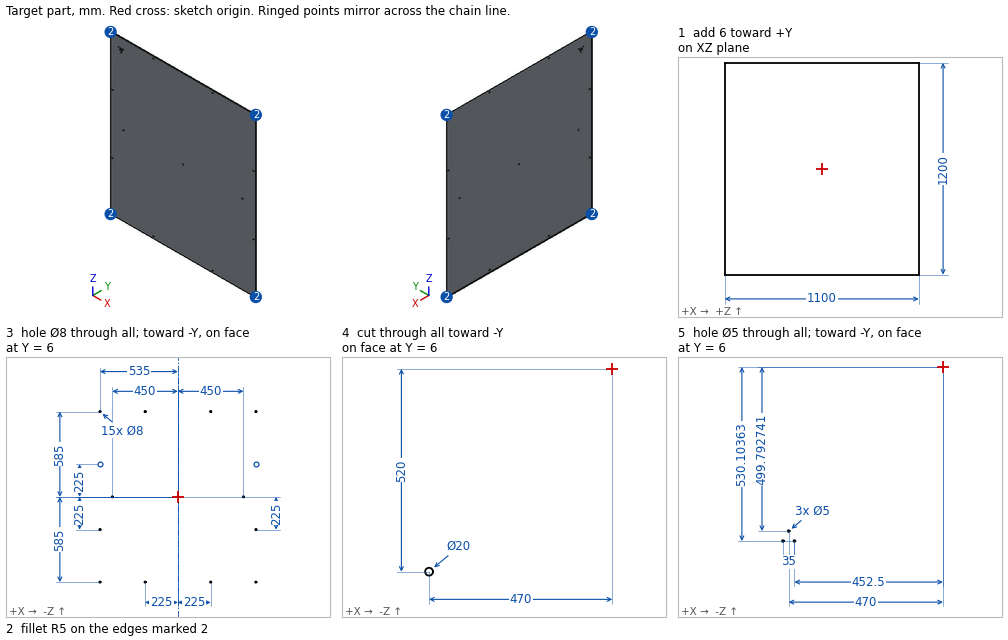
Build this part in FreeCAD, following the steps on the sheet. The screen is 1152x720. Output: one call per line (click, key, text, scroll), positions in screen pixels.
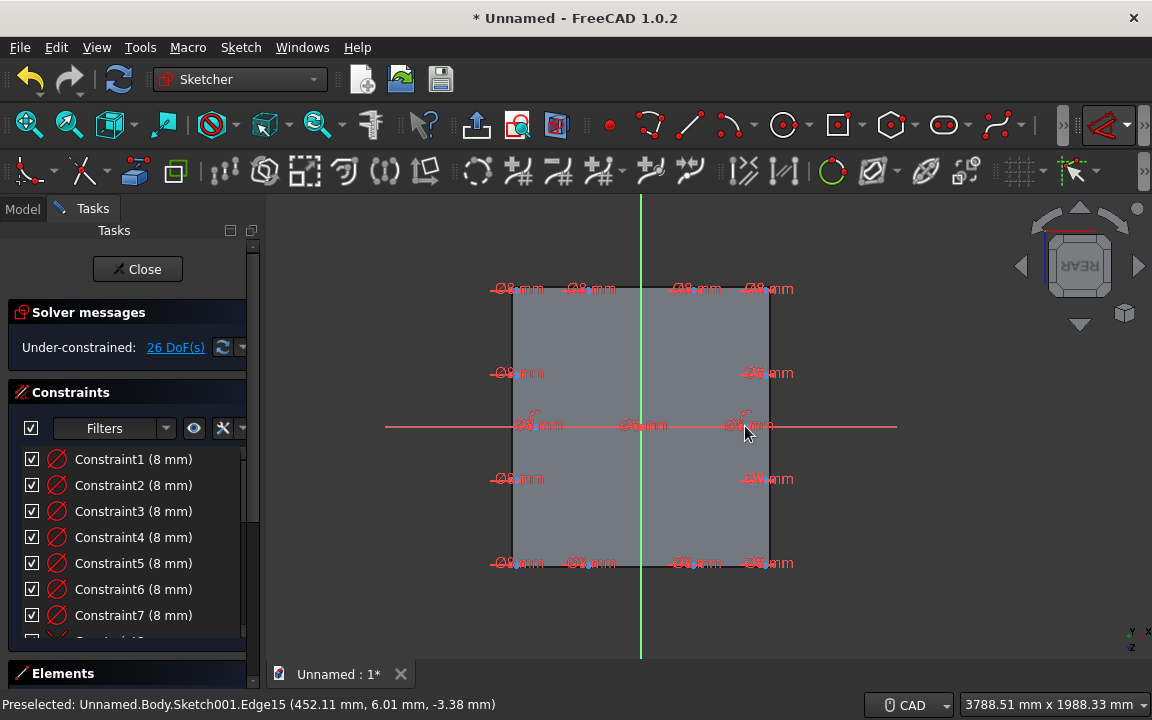
click(516, 291)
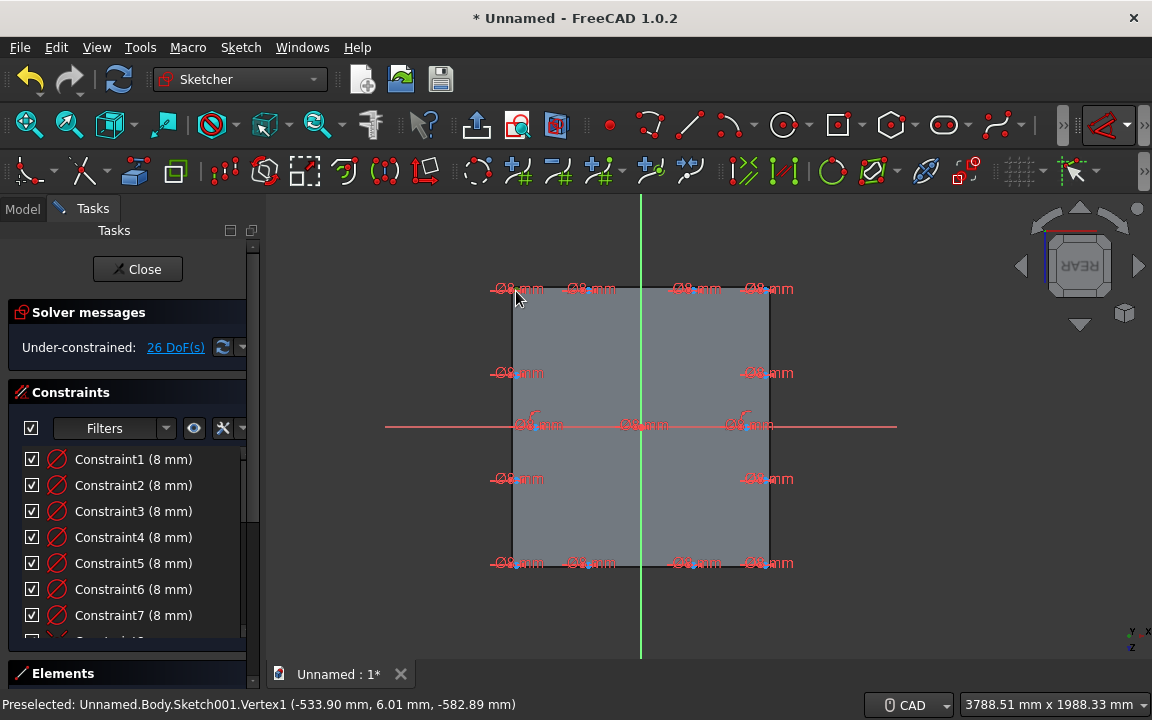
click(766, 291)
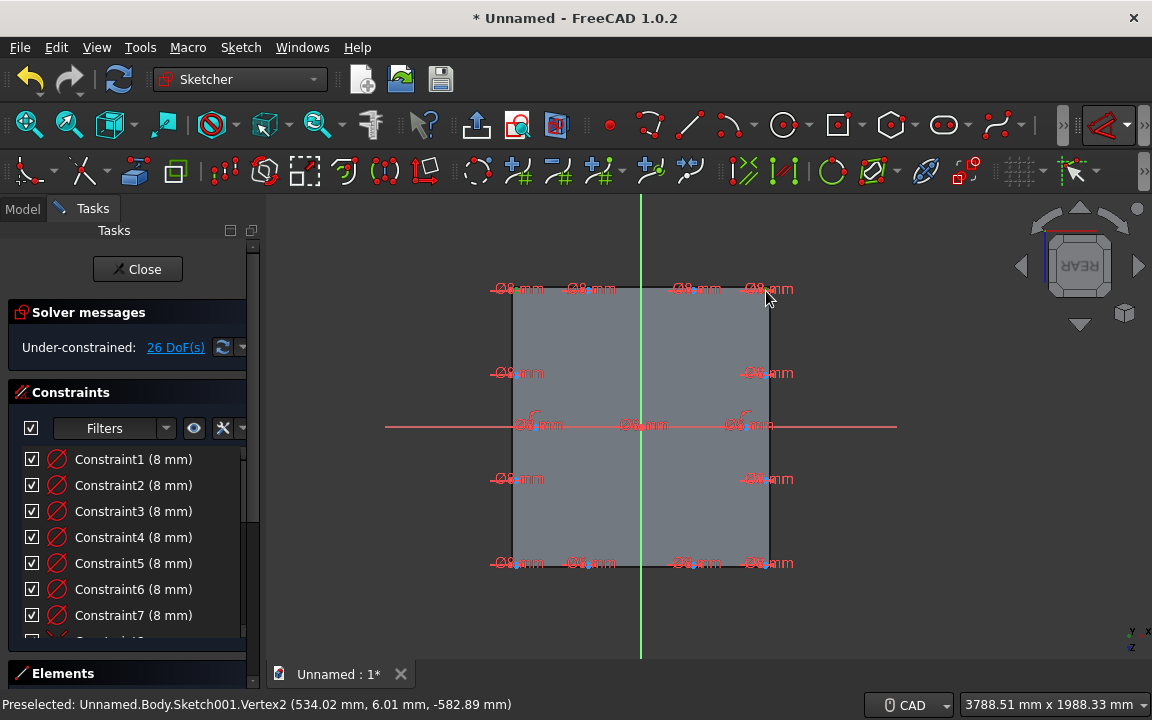
key(h)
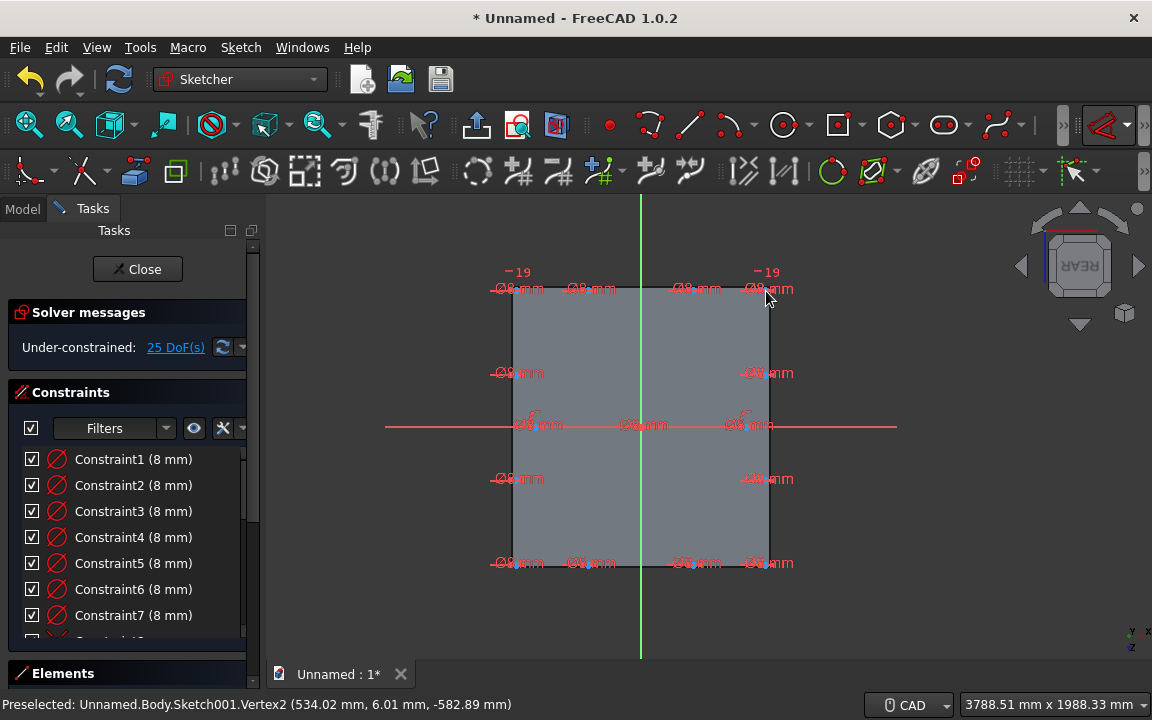
click(516, 291)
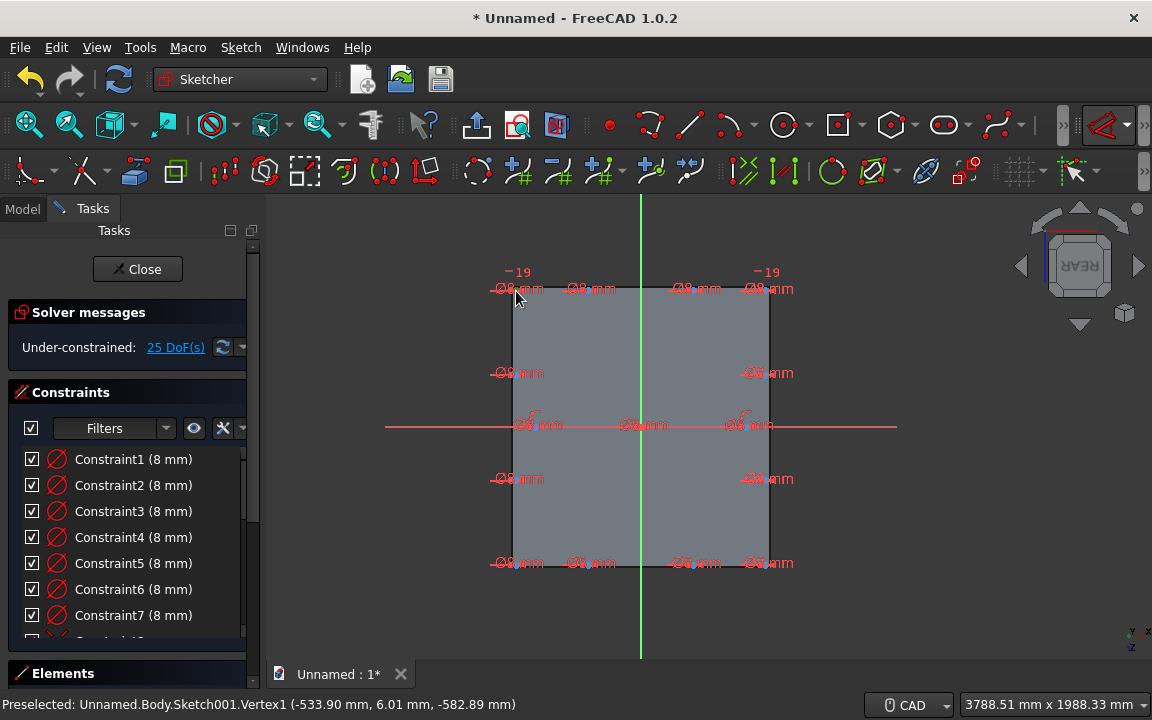
click(516, 565)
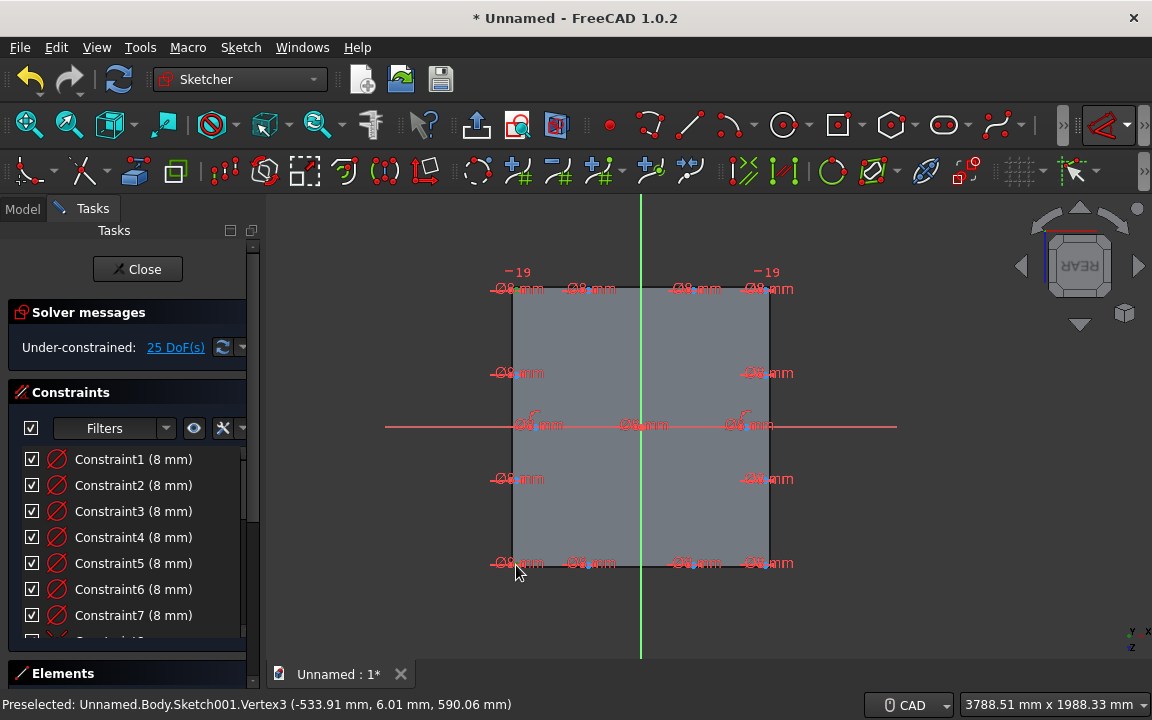
key(v)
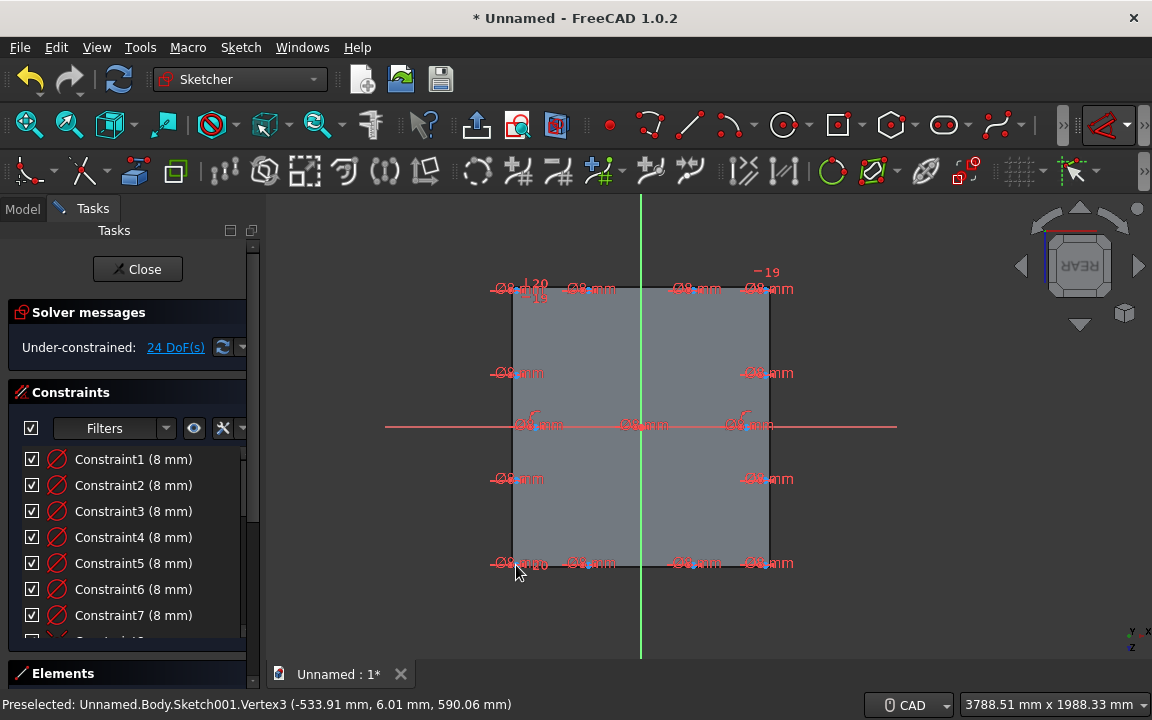
click(766, 291)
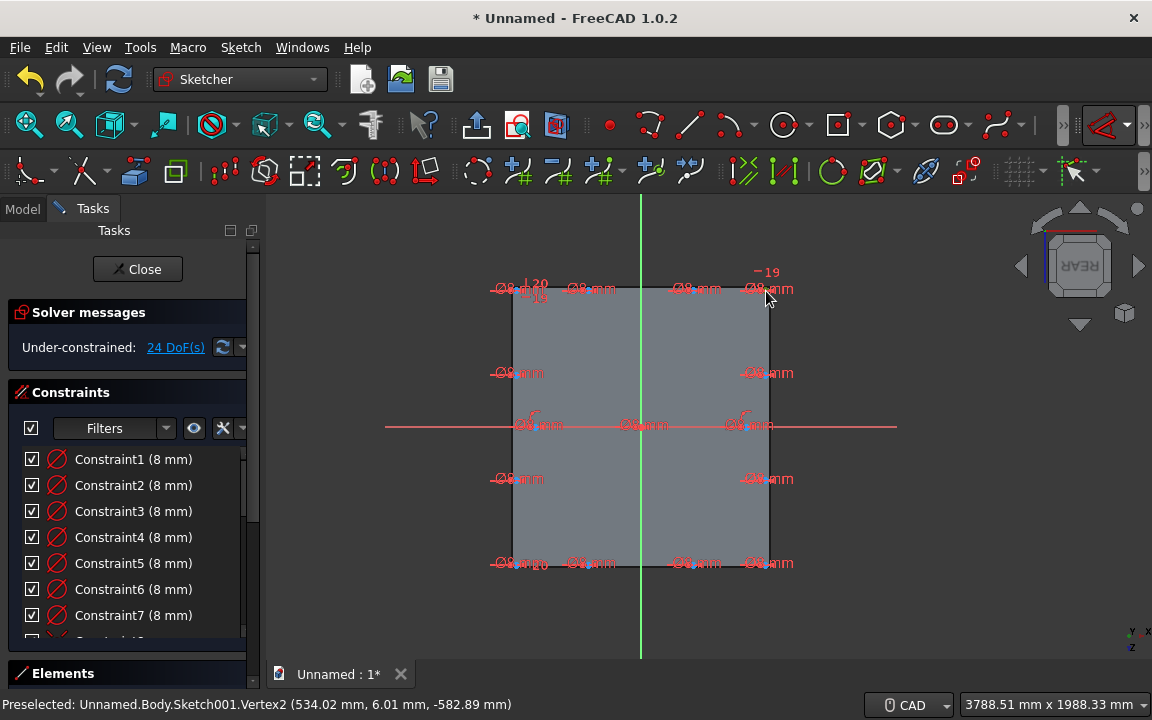
click(766, 565)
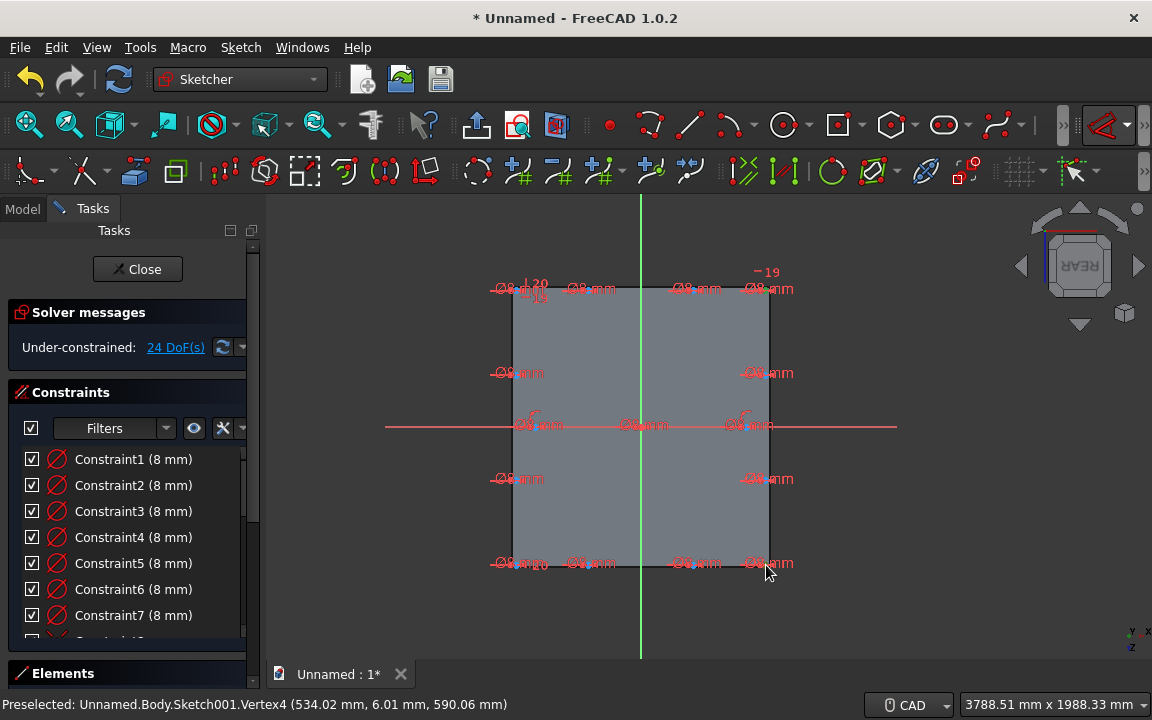
key(v)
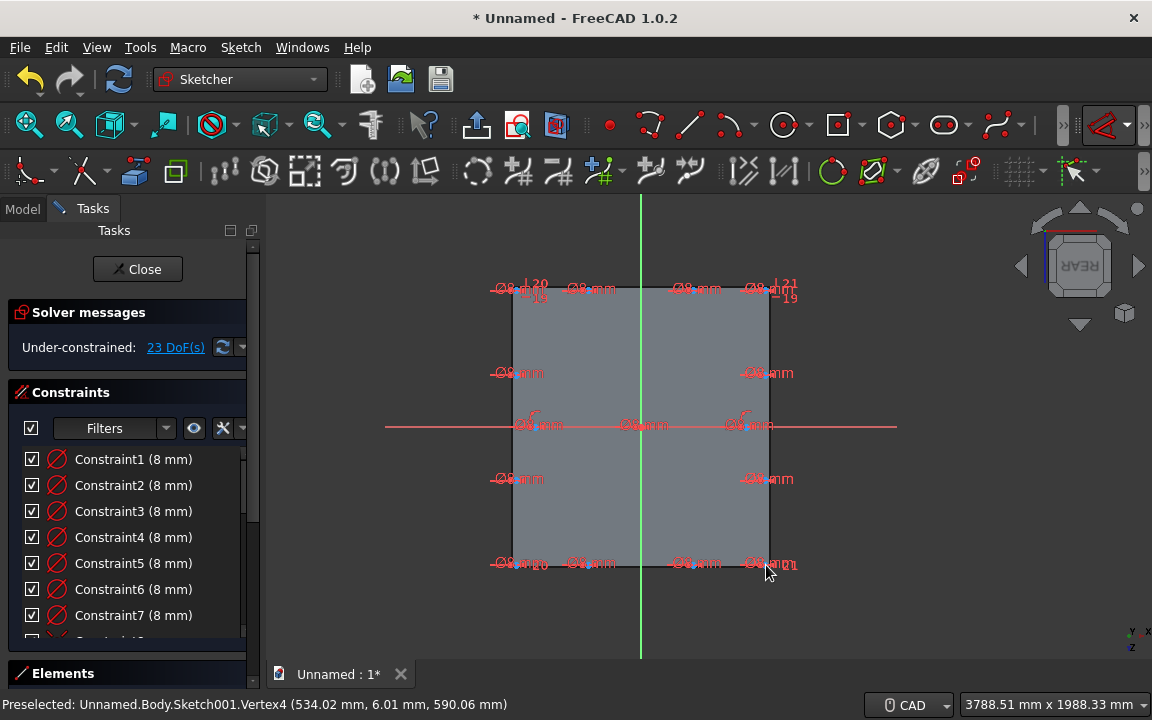
click(516, 565)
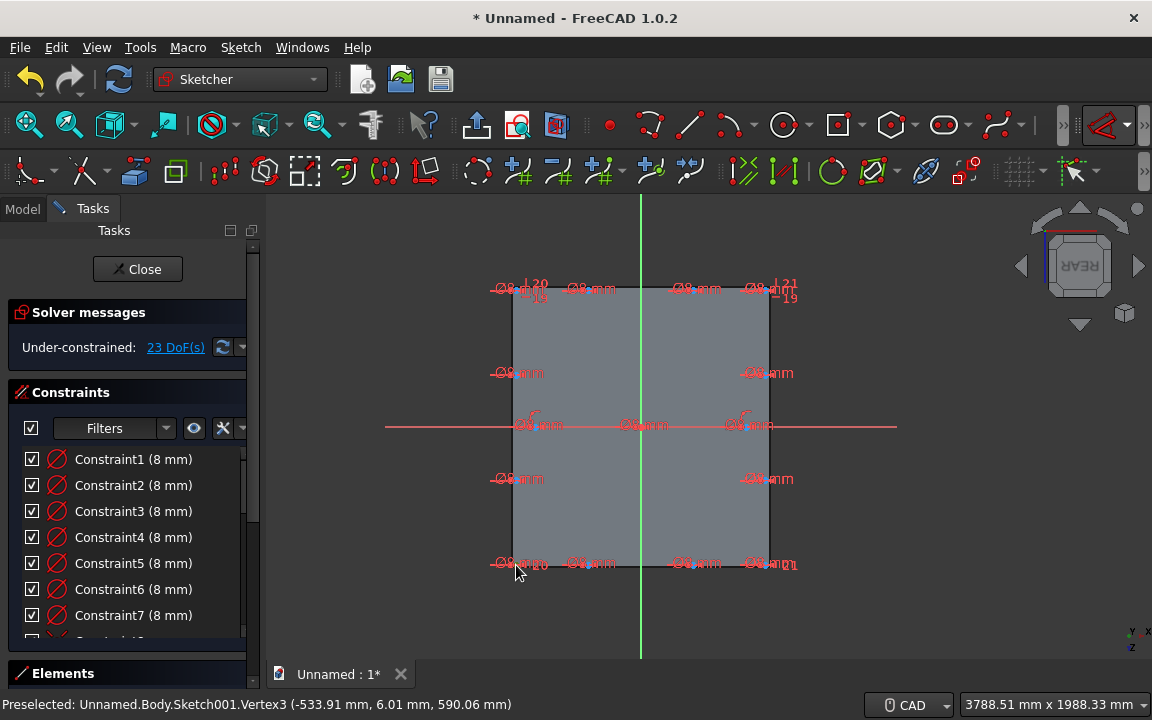
click(766, 565)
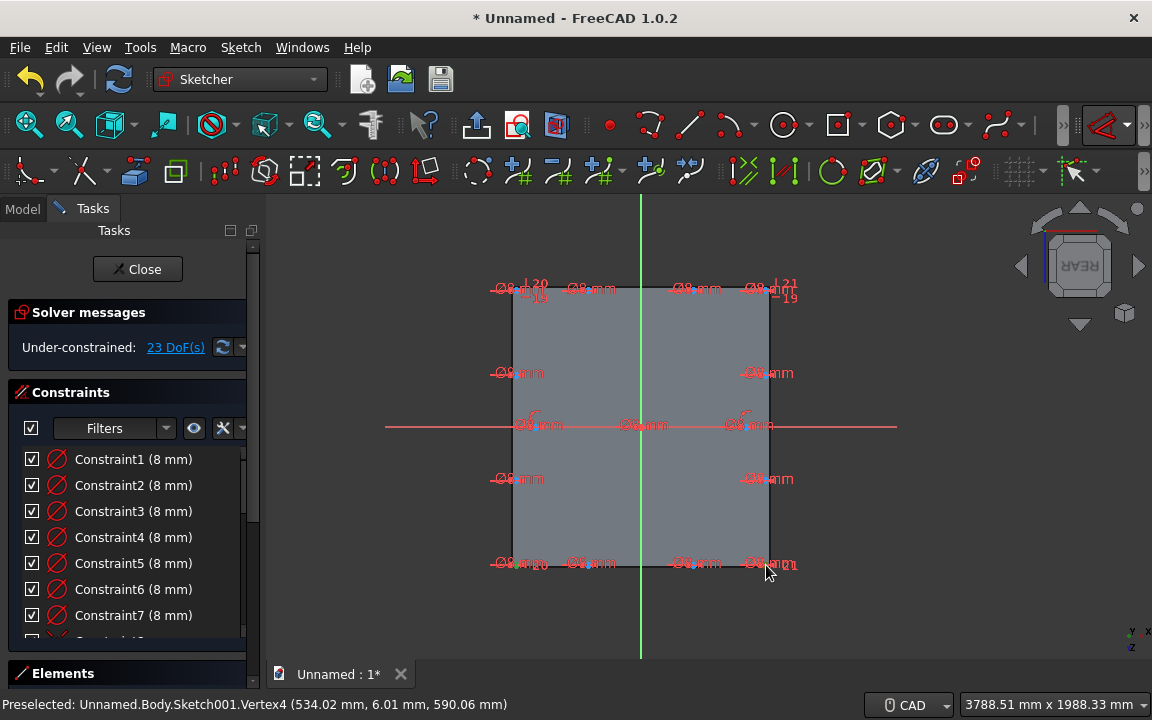
key(h)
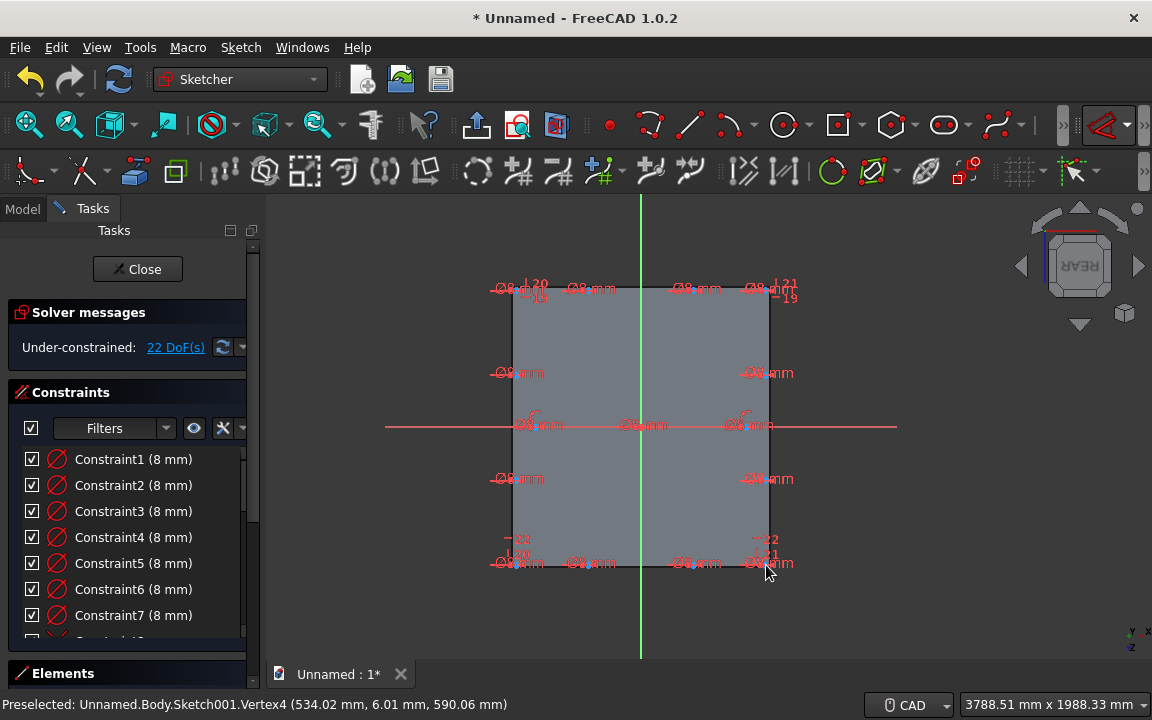
click(516, 565)